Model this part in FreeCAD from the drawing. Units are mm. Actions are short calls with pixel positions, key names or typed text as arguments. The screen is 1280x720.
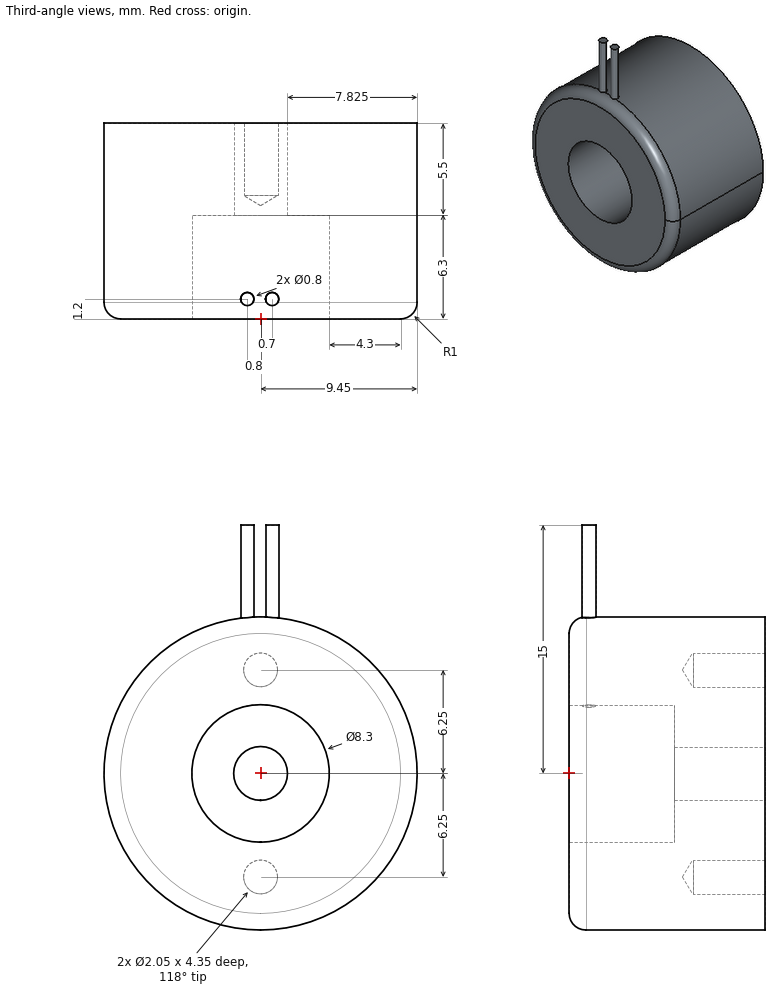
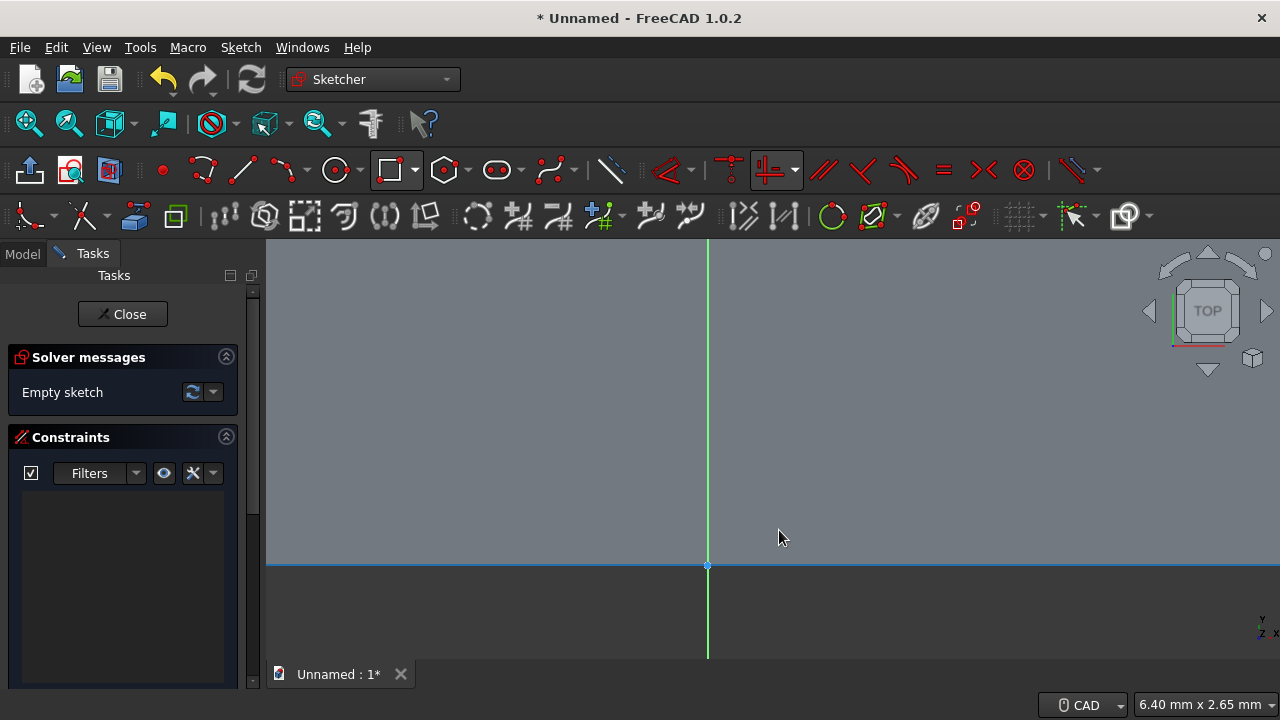
click(336, 170)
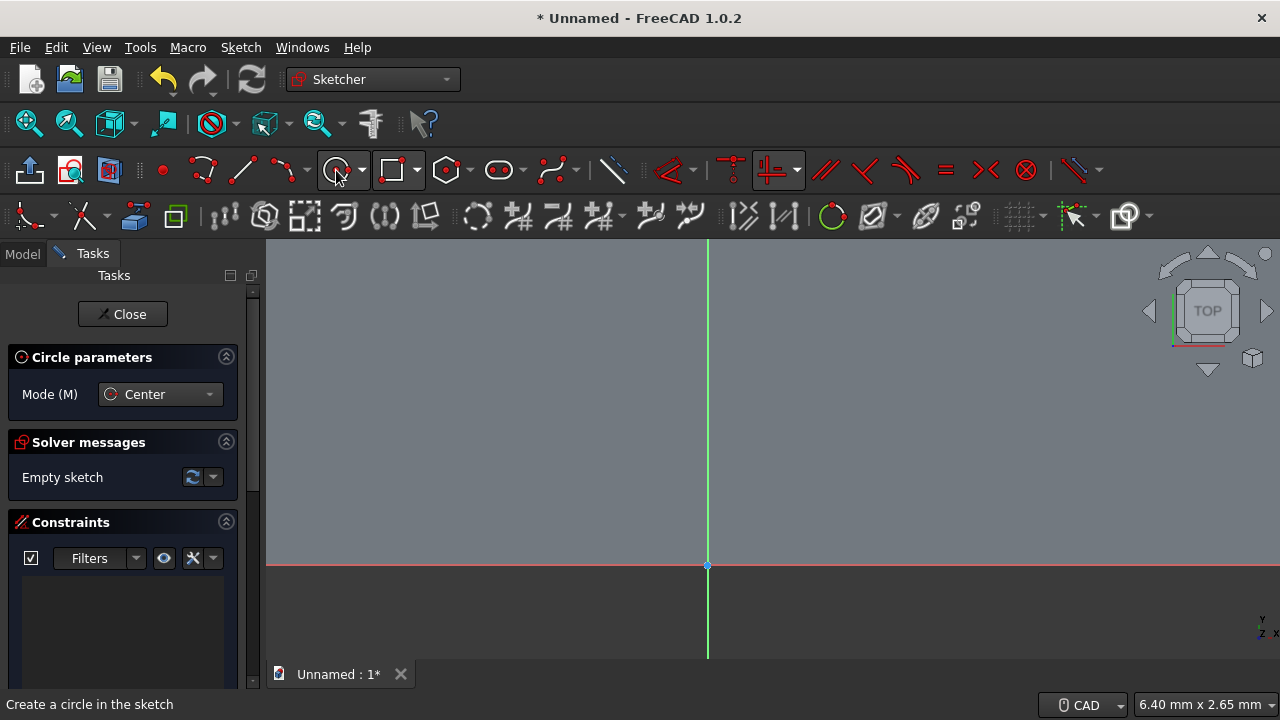
click(581, 375)
move(626, 330)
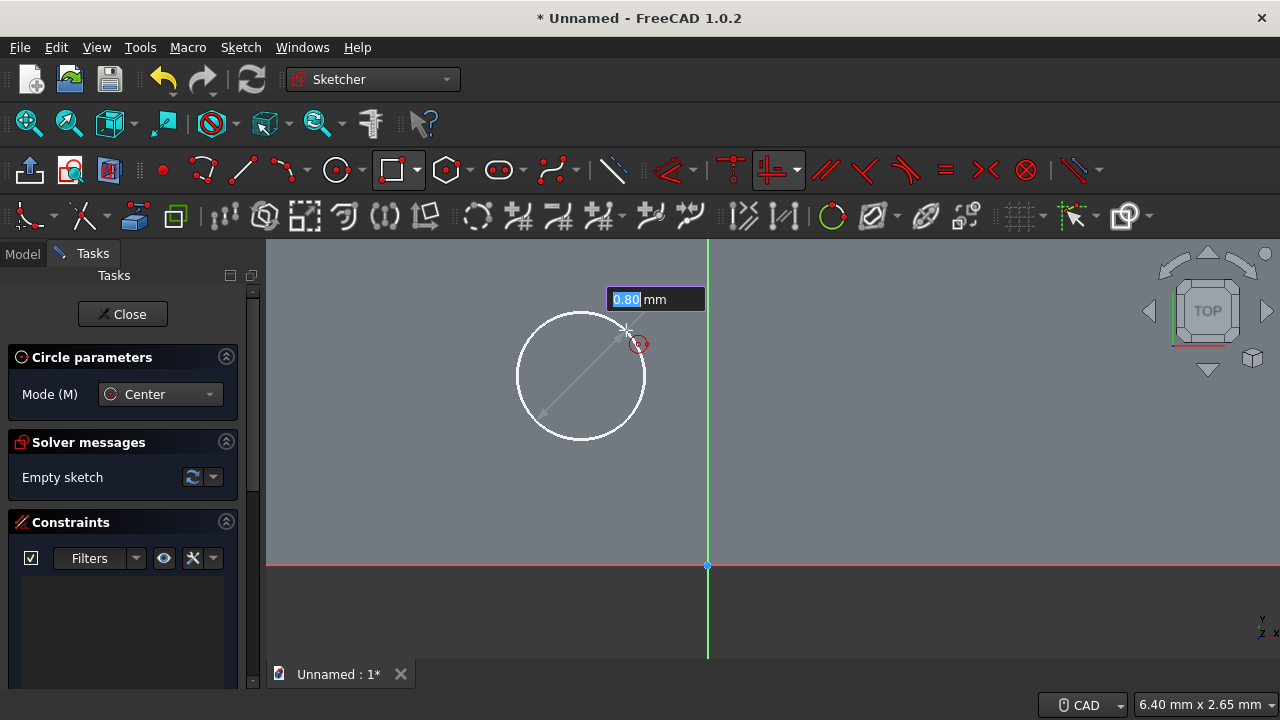
text(0.8)
key(Return)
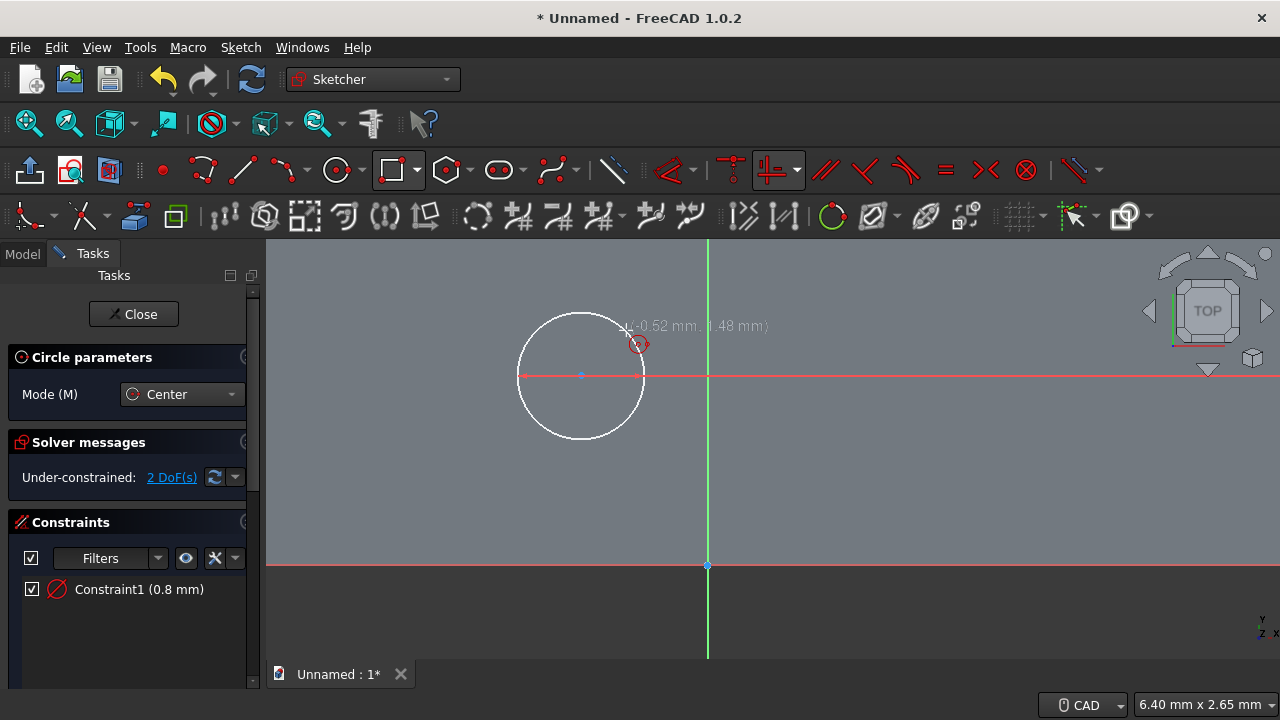
click(819, 375)
move(864, 330)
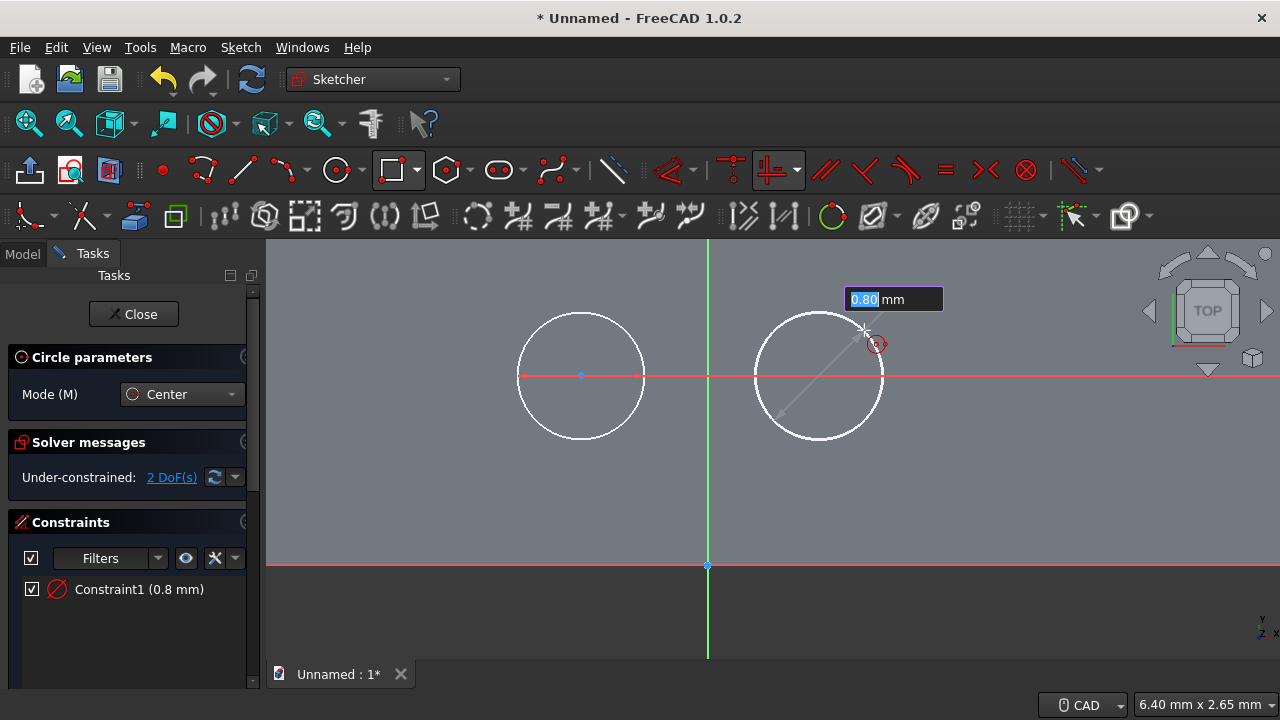
text(0.8)
key(Return)
key(Escape)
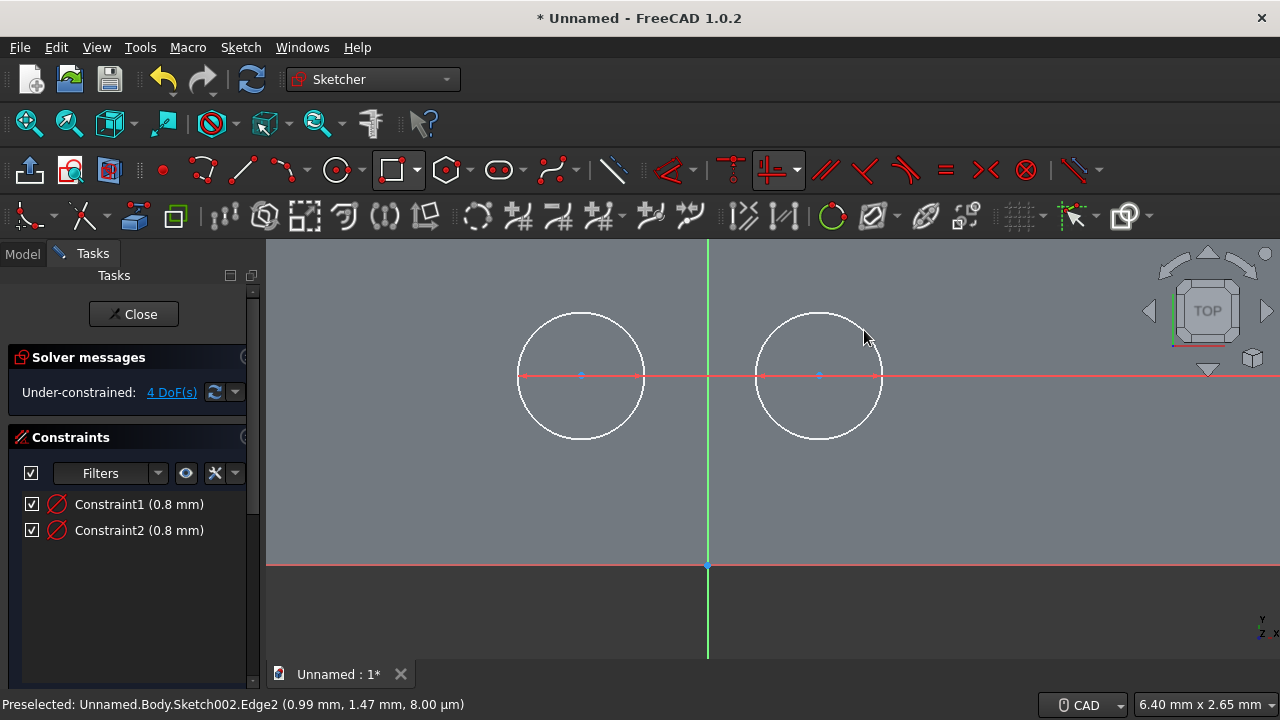
click(581, 376)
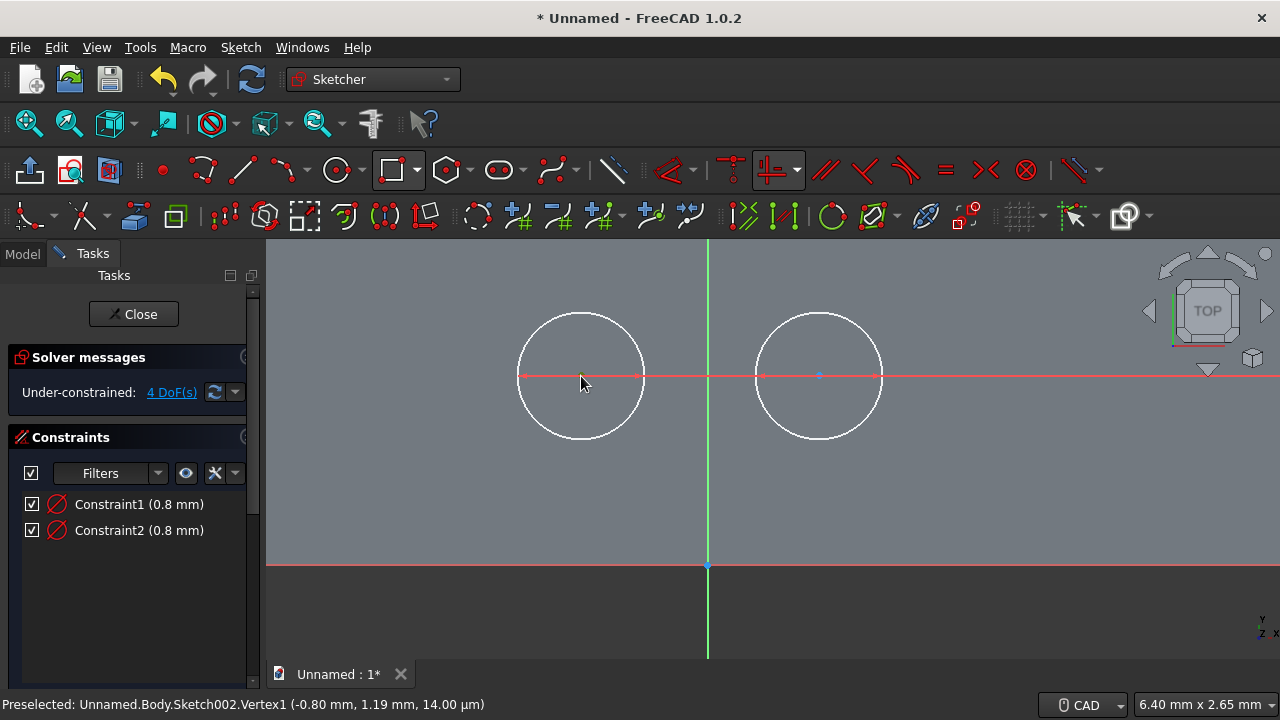
click(819, 376)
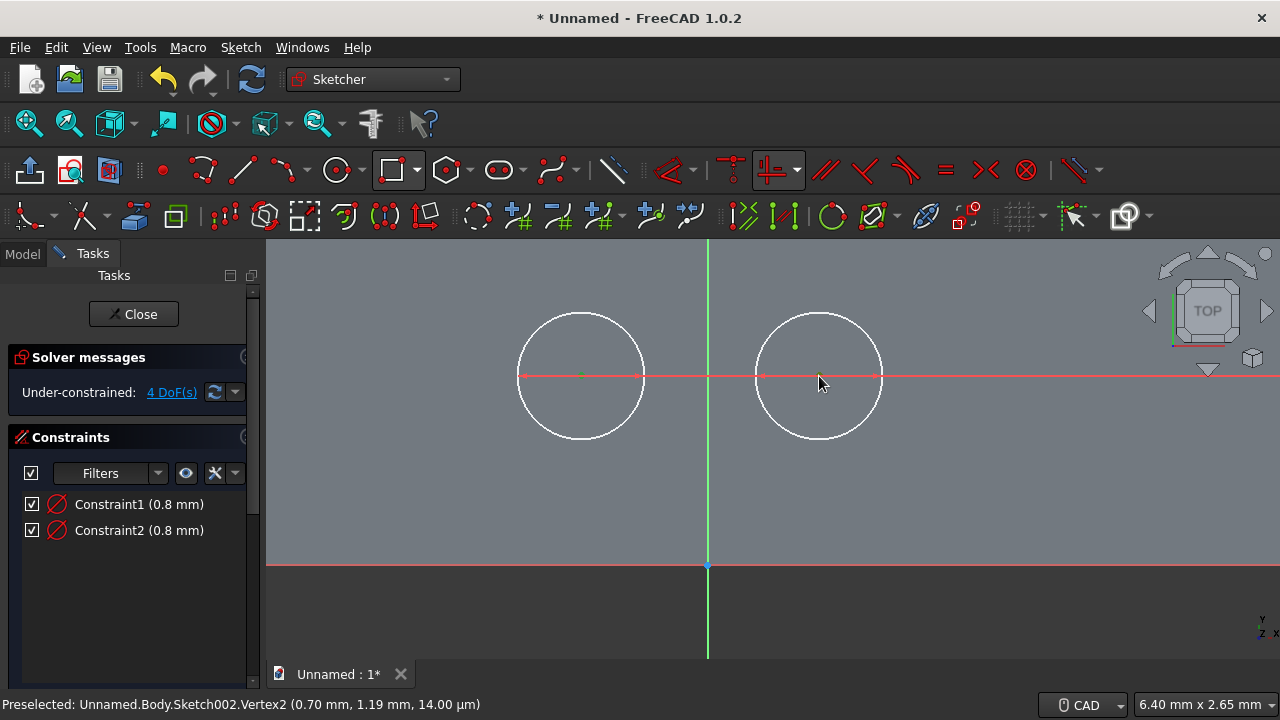
key(h)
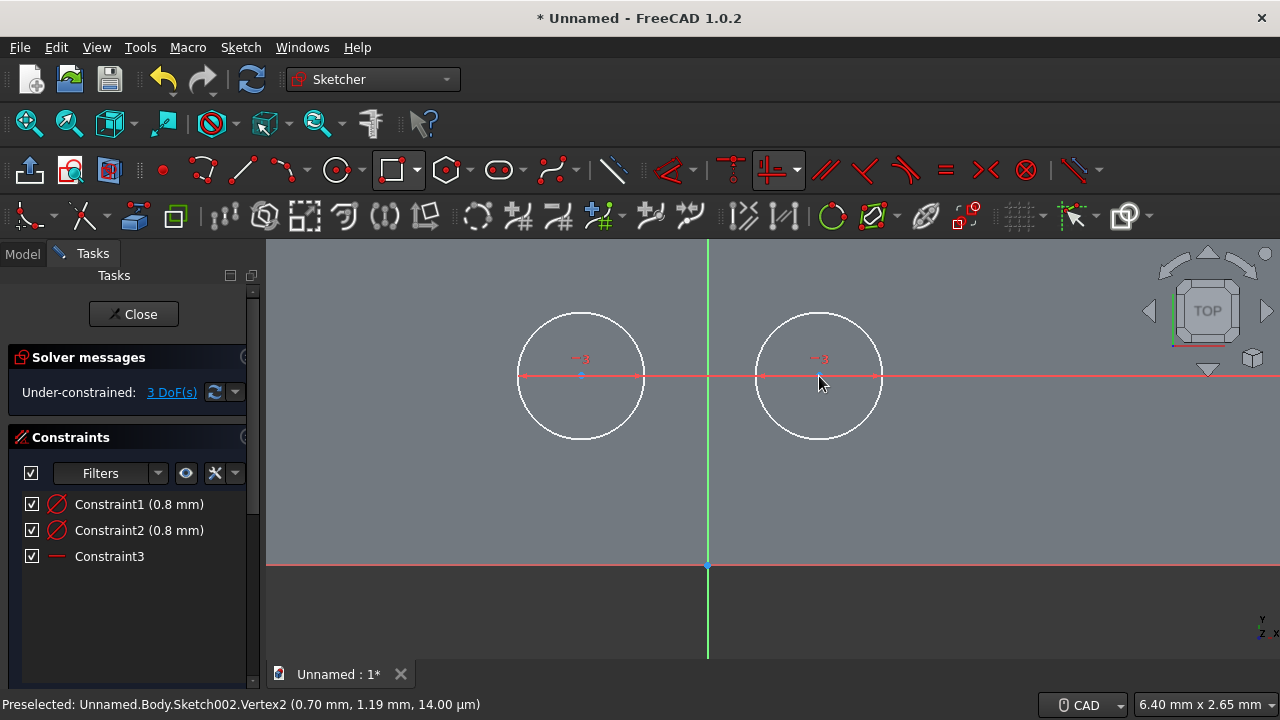
key(d)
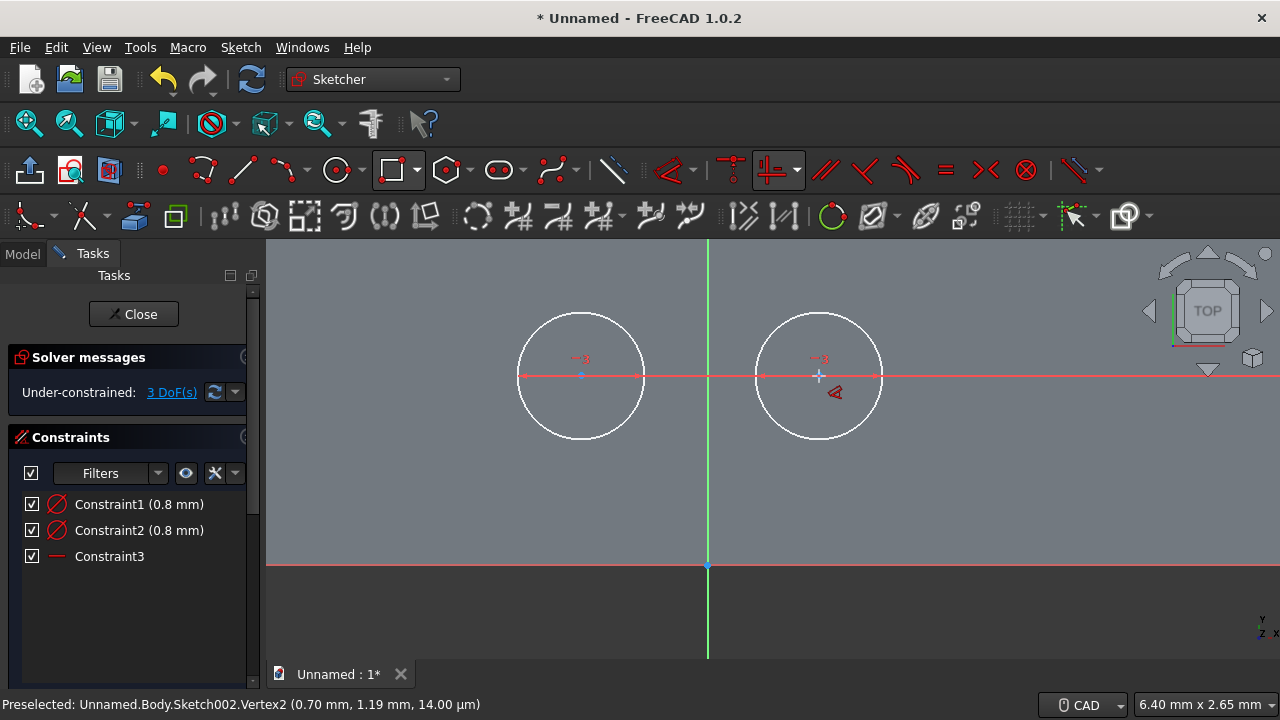
click(581, 376)
click(644, 599)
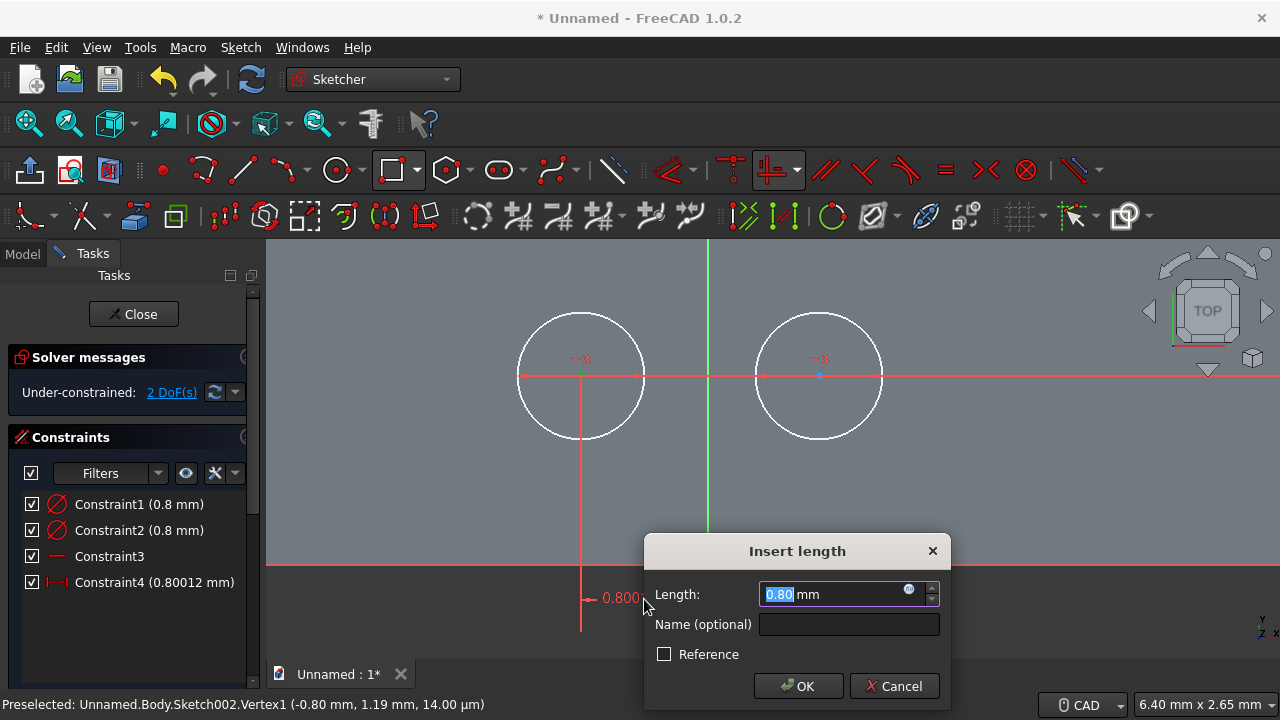
text(0.8)
key(Return)